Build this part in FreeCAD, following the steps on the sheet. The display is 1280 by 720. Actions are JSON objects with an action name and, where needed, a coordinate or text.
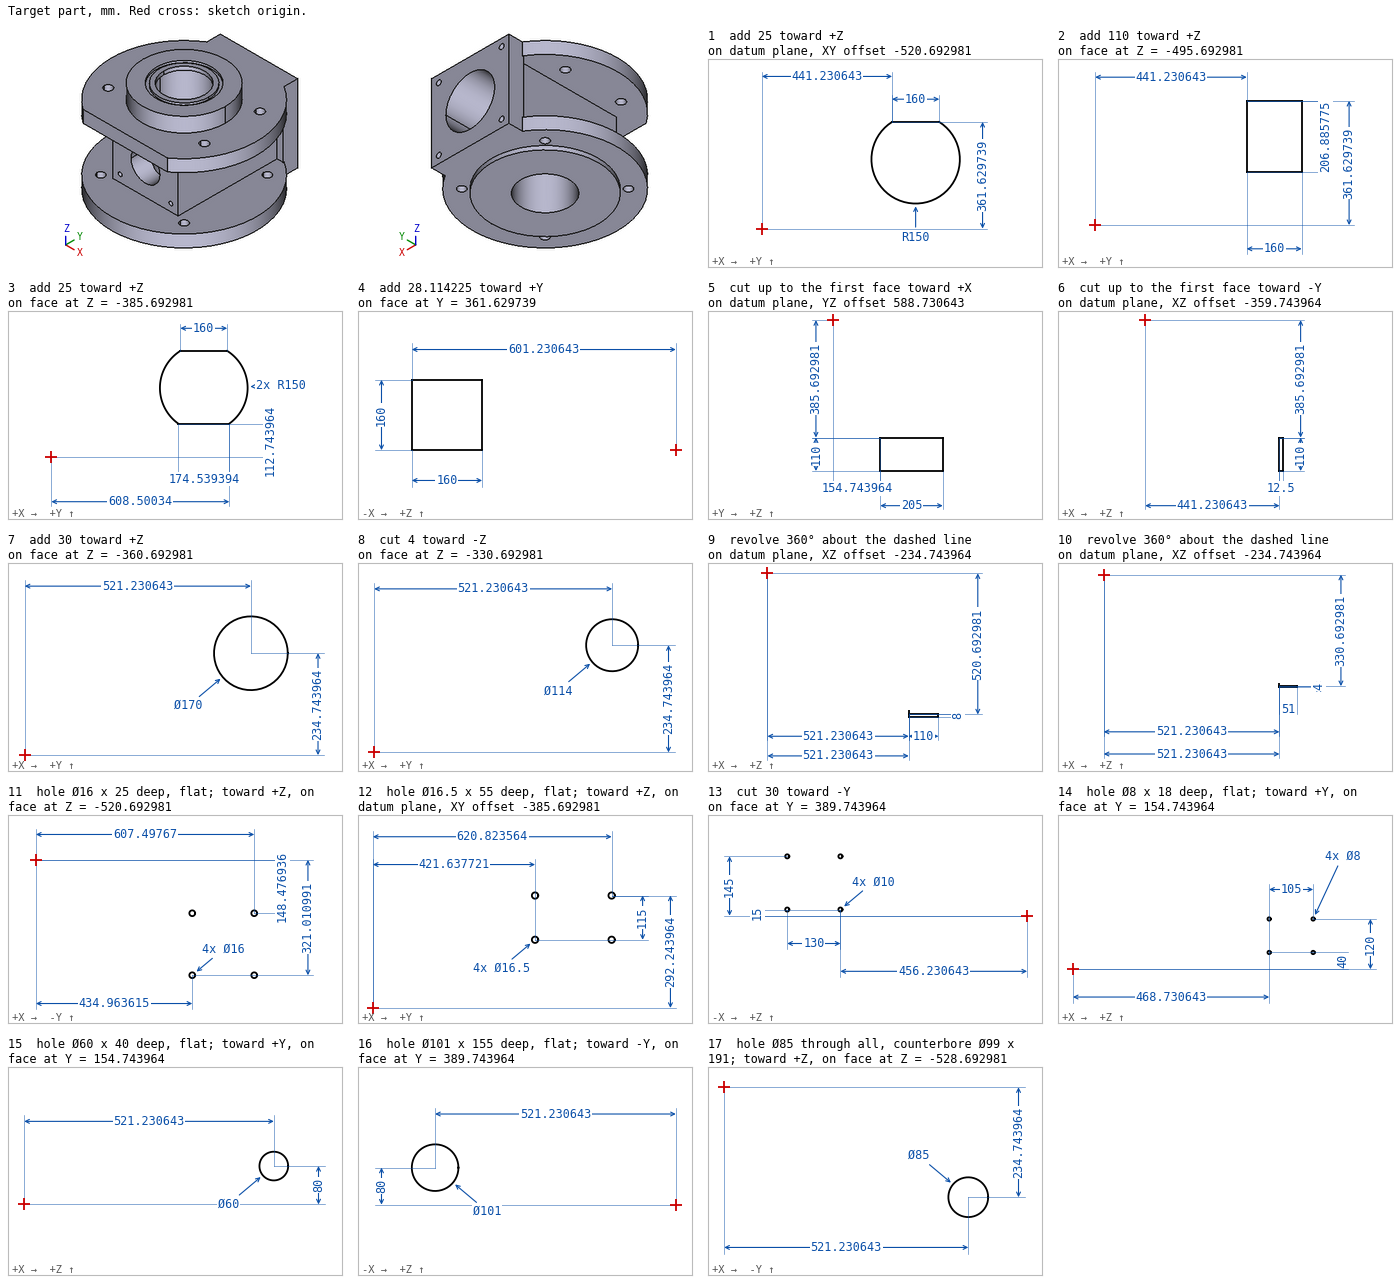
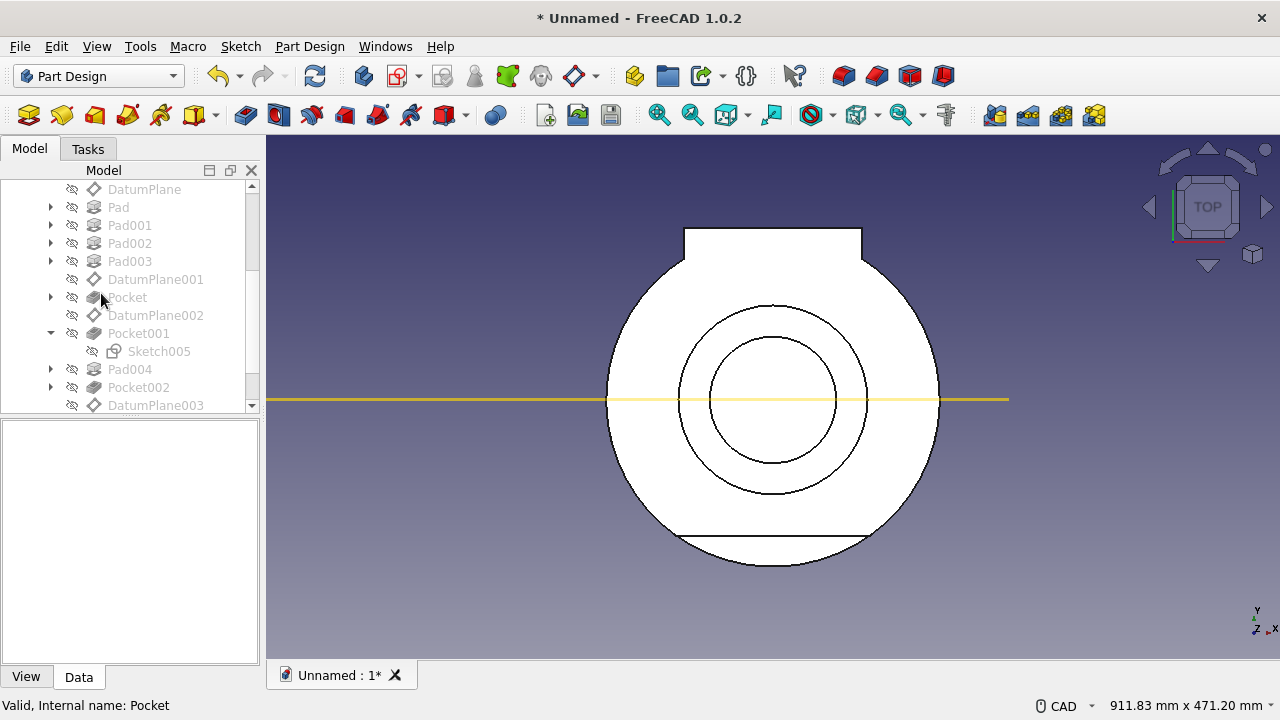
{"action": "scroll", "coordinate": [141, 293], "scroll_direction": "up", "scroll_amount": 15}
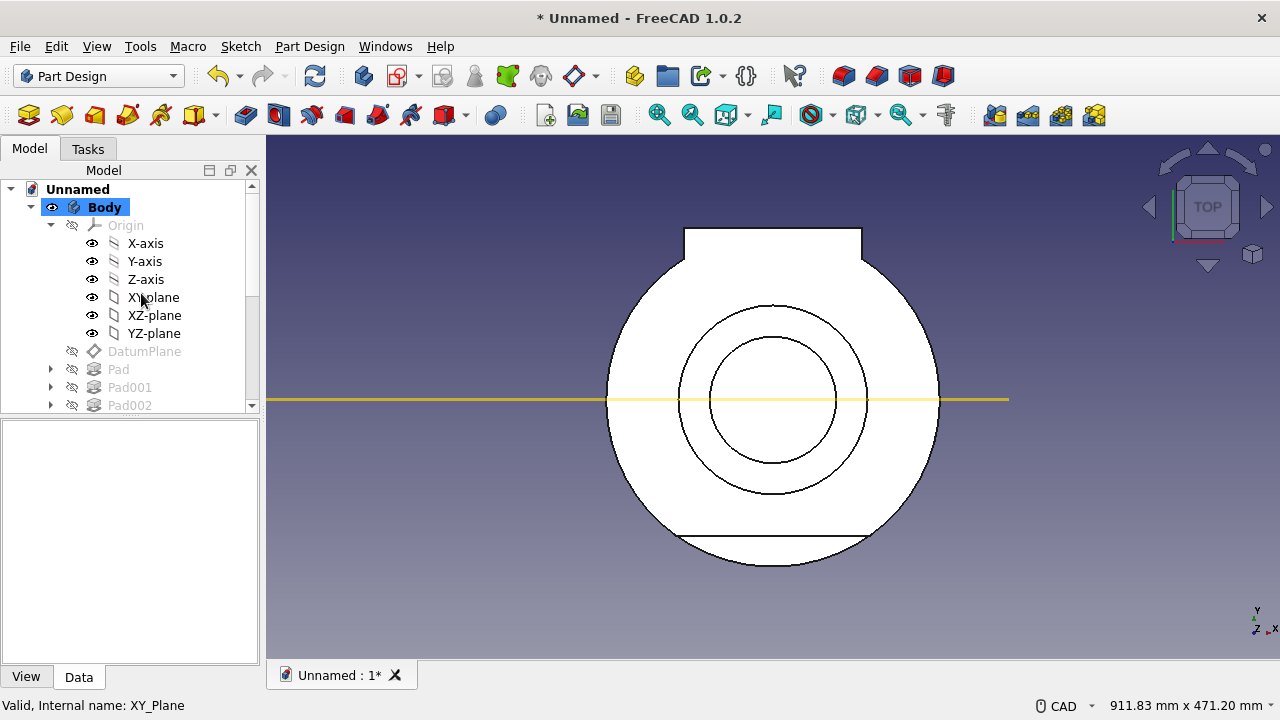
{"action": "scroll", "coordinate": [101, 293], "scroll_direction": "down", "scroll_amount": 6}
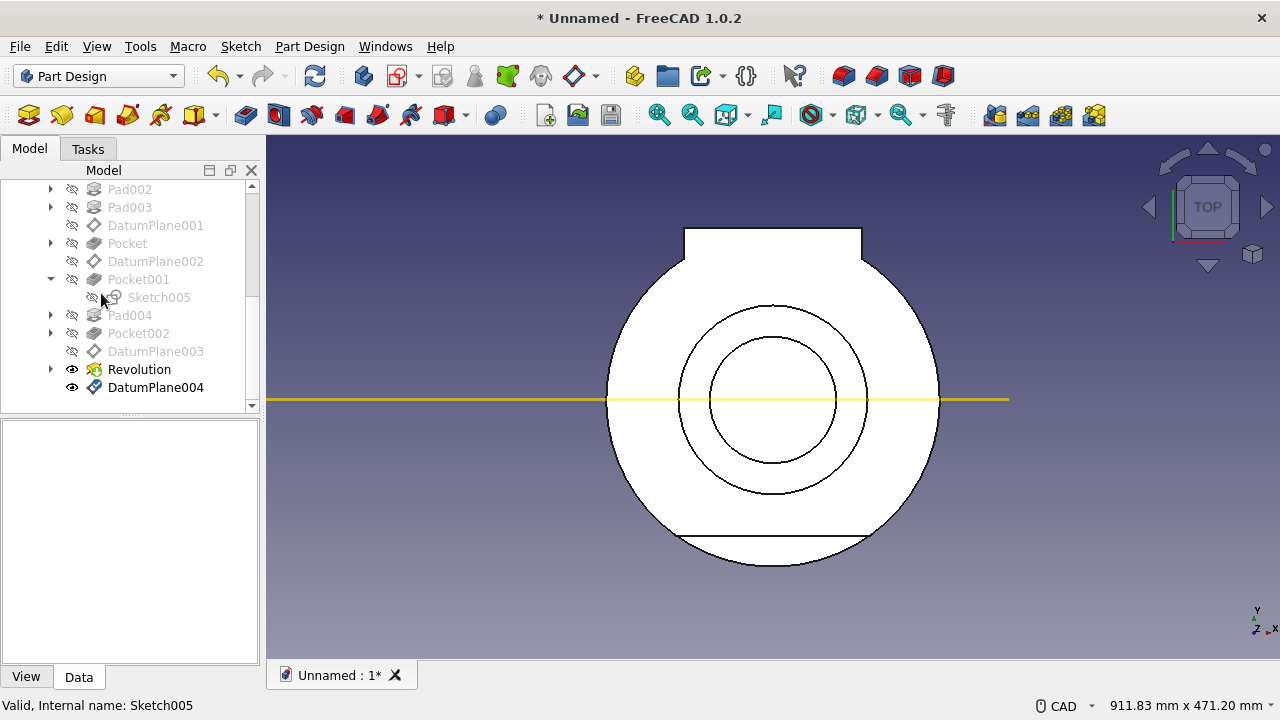
{"action": "left_click", "coordinate": [117, 387]}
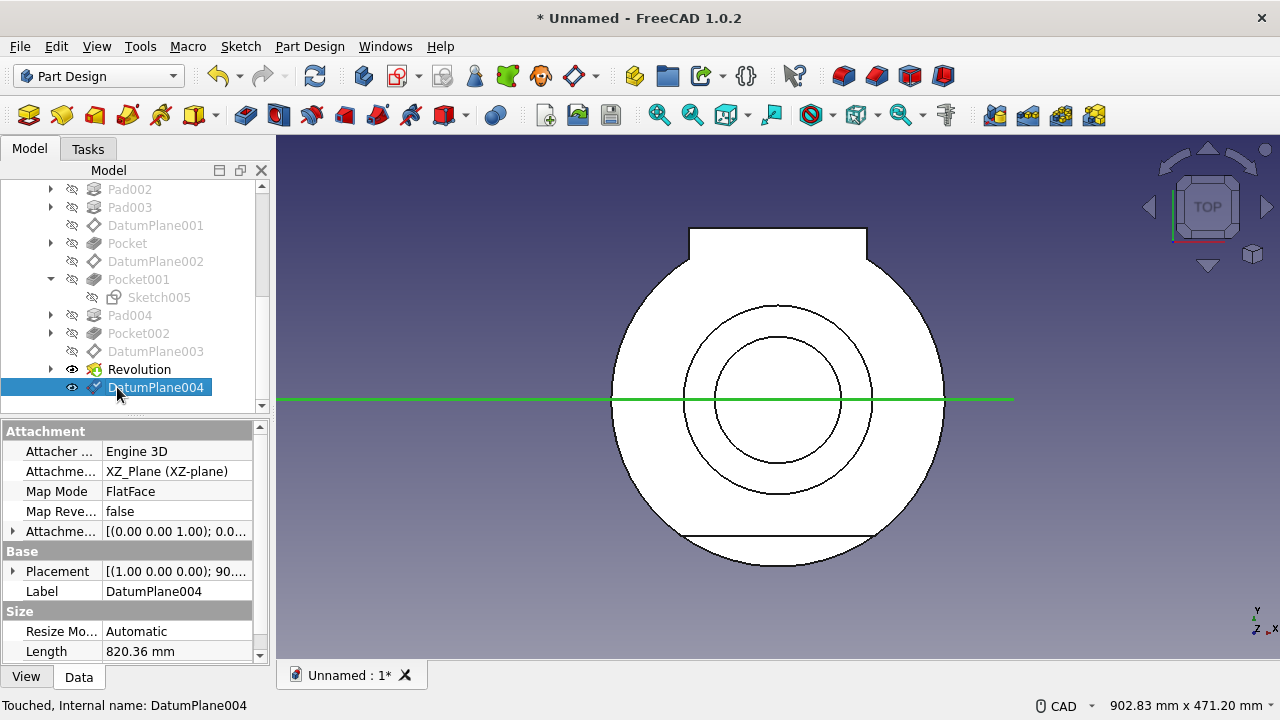
{"action": "left_click", "coordinate": [396, 76]}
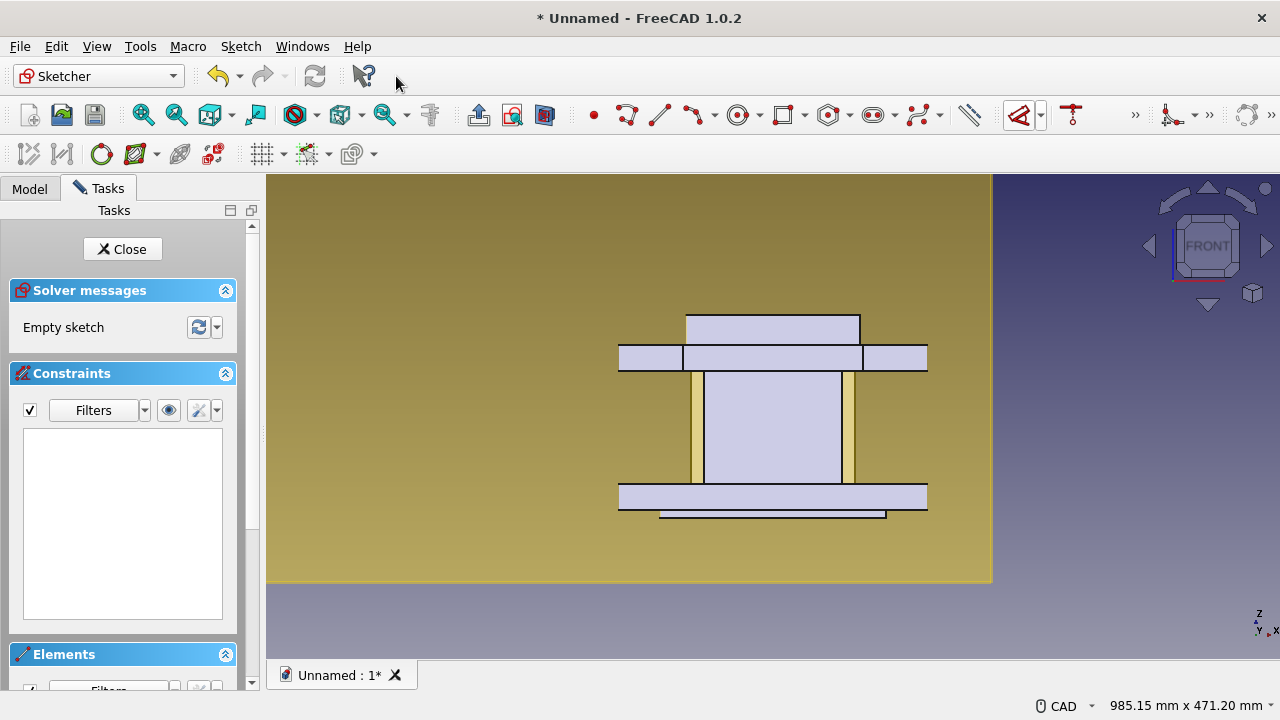
{"action": "left_click", "coordinate": [545, 116]}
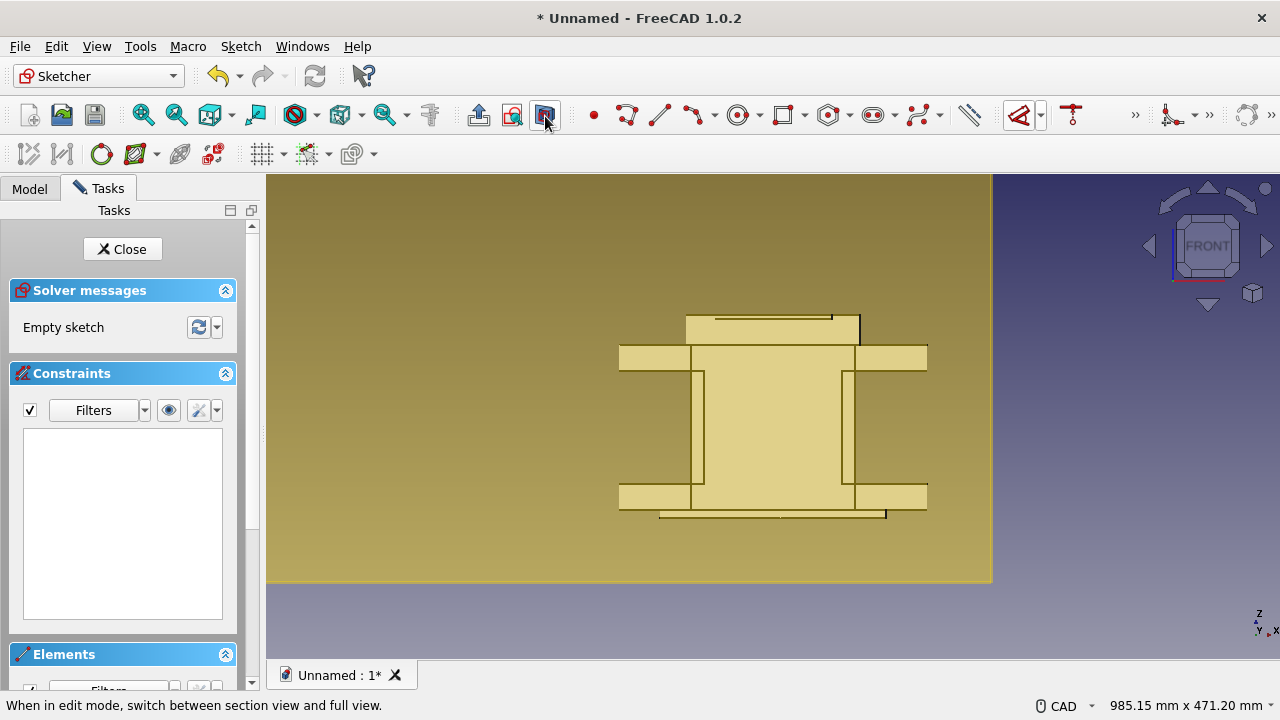
{"action": "scroll", "coordinate": [809, 302], "scroll_direction": "up", "scroll_amount": 12}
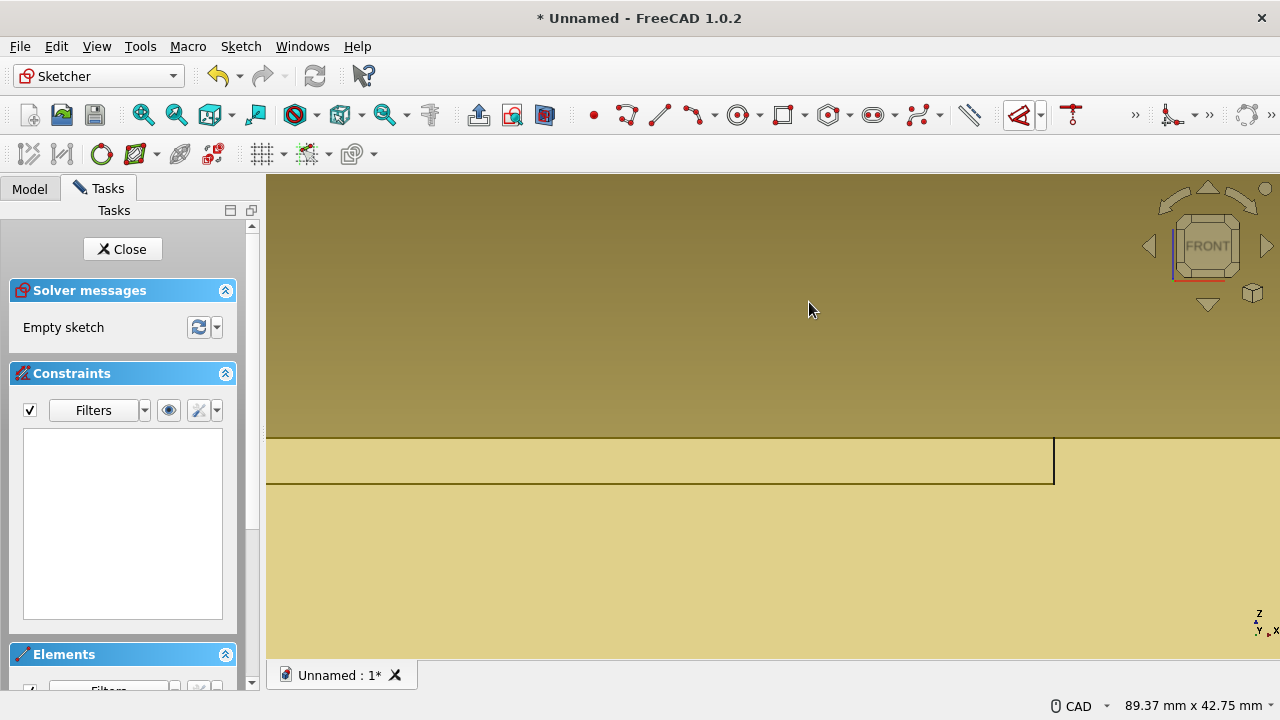
{"action": "left_click", "coordinate": [782, 116]}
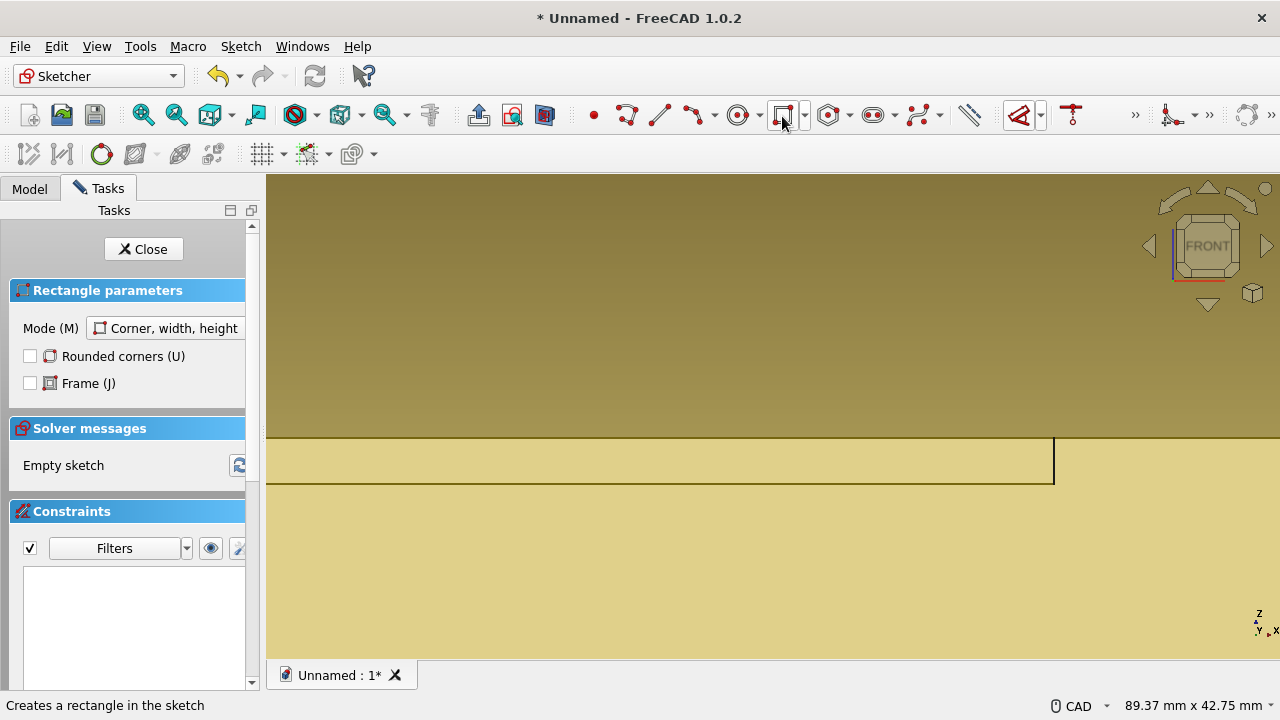
{"action": "left_click", "coordinate": [407, 438]}
{"action": "left_click", "coordinate": [985, 484]}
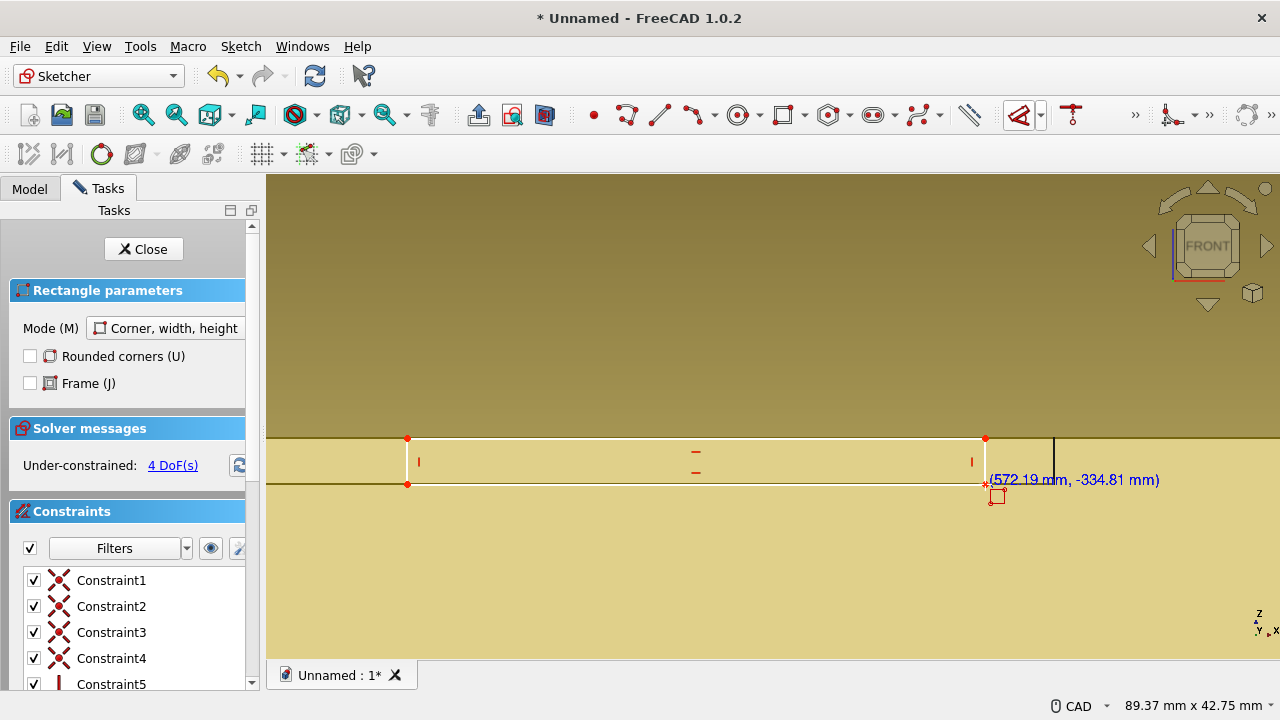
{"action": "left_click", "coordinate": [660, 116]}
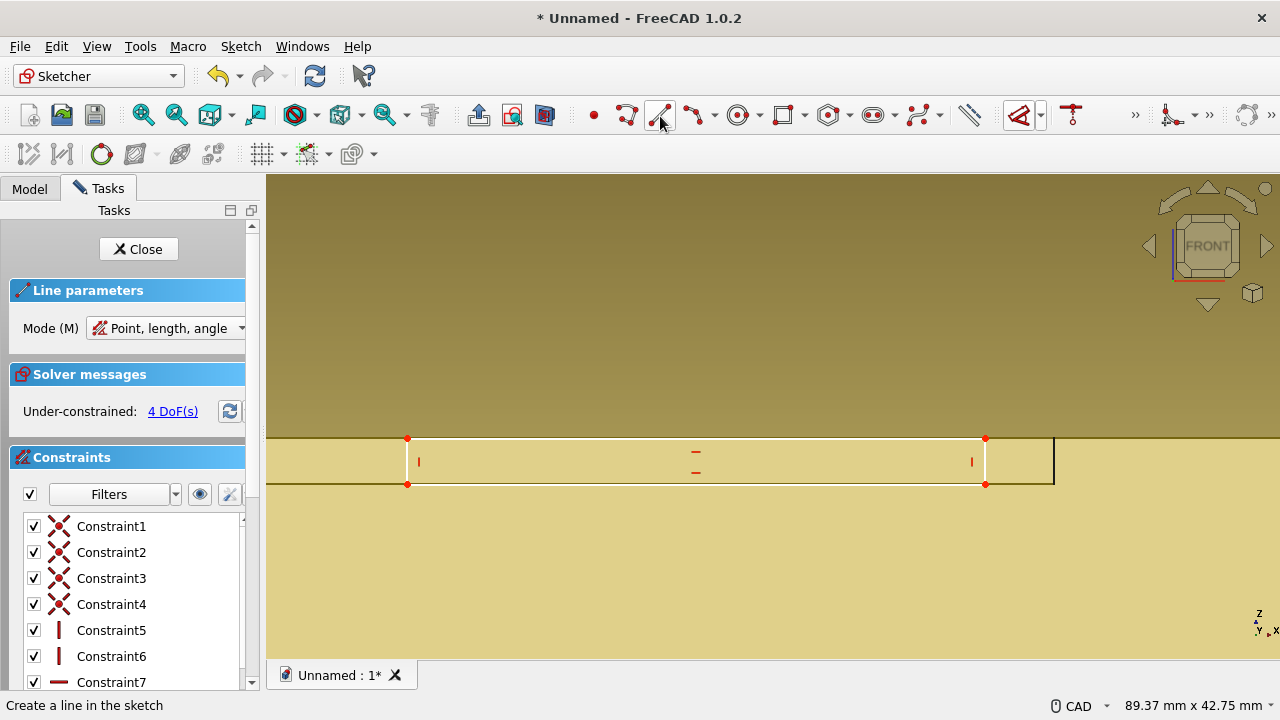
{"action": "left_click", "coordinate": [407, 415]}
{"action": "left_click", "coordinate": [407, 346]}
{"action": "key", "text": "Escape"}